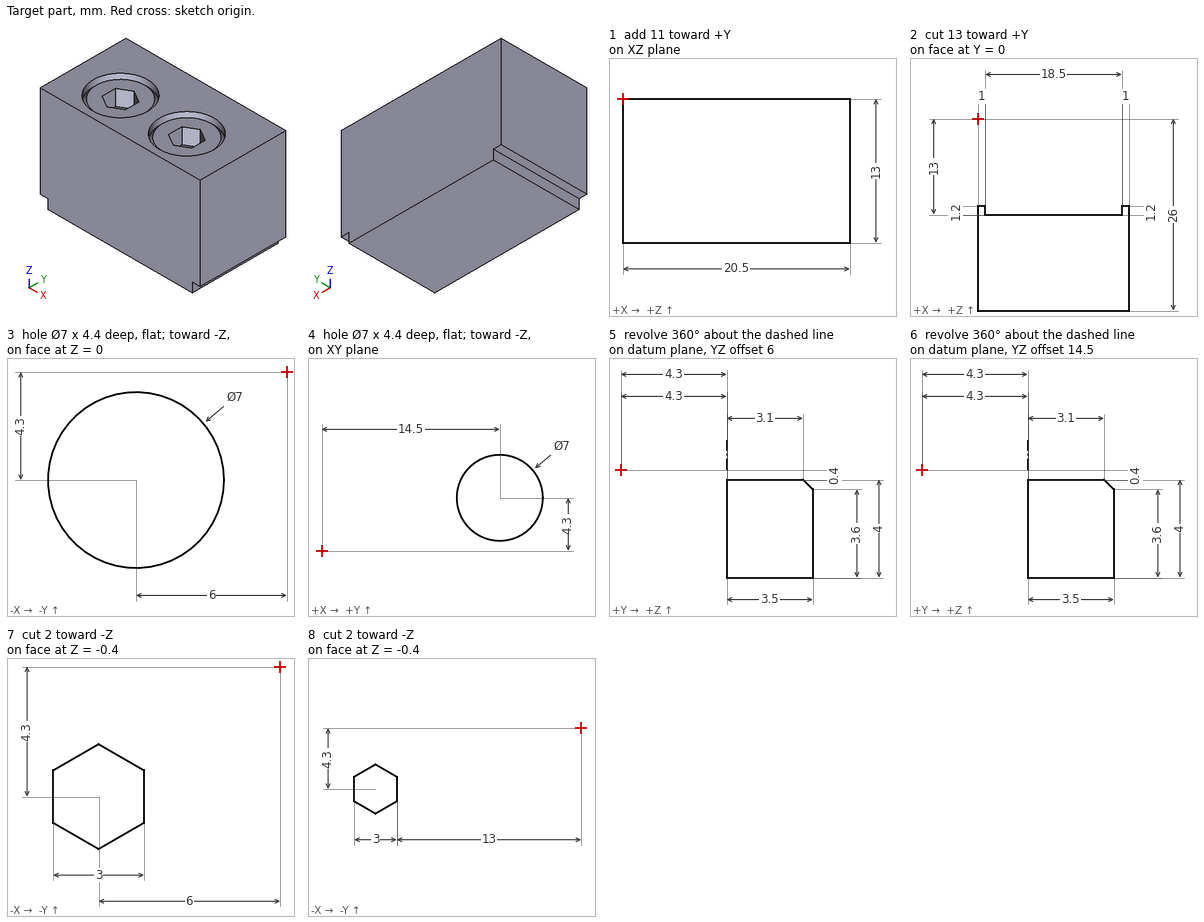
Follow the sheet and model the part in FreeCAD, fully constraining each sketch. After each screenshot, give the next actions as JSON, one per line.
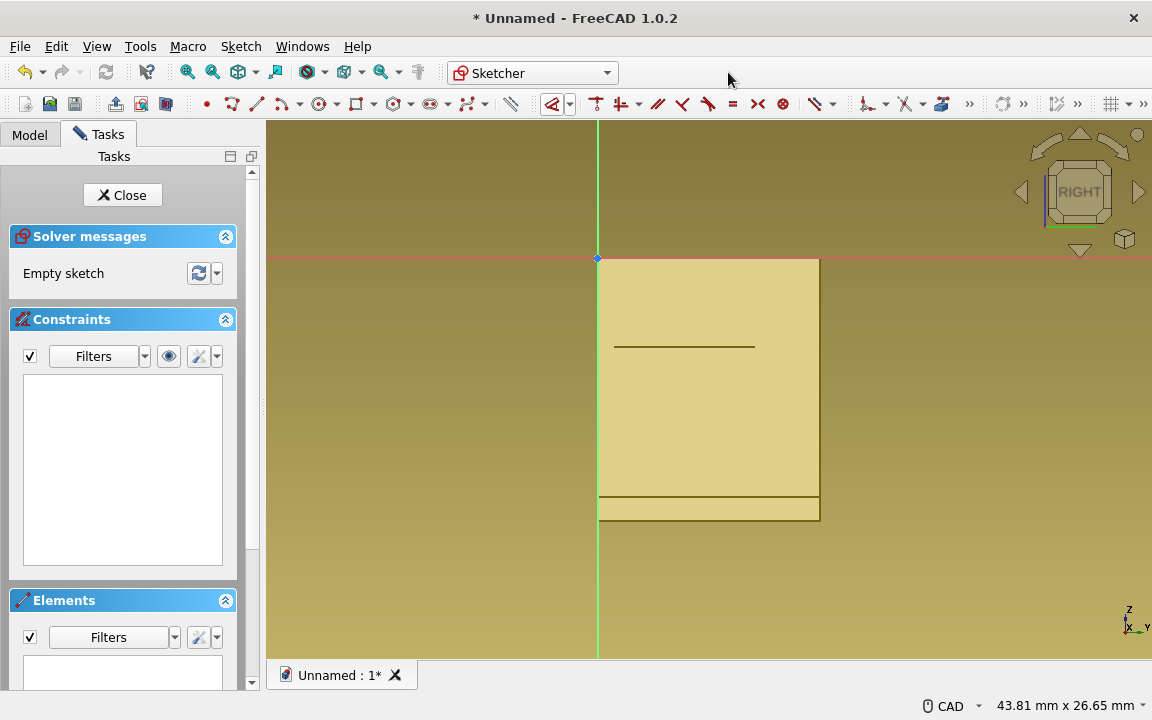
{"action": "scroll", "coordinate": [692, 248], "scroll_direction": "up", "scroll_amount": 6}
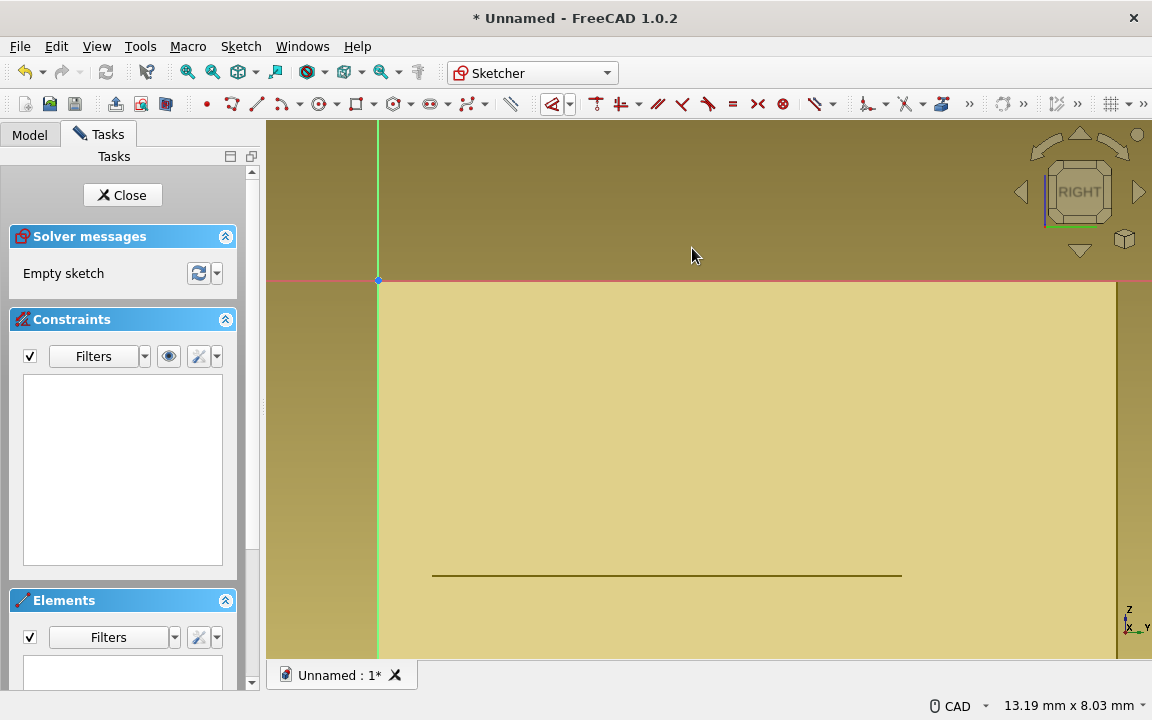
{"action": "left_click", "coordinate": [232, 104]}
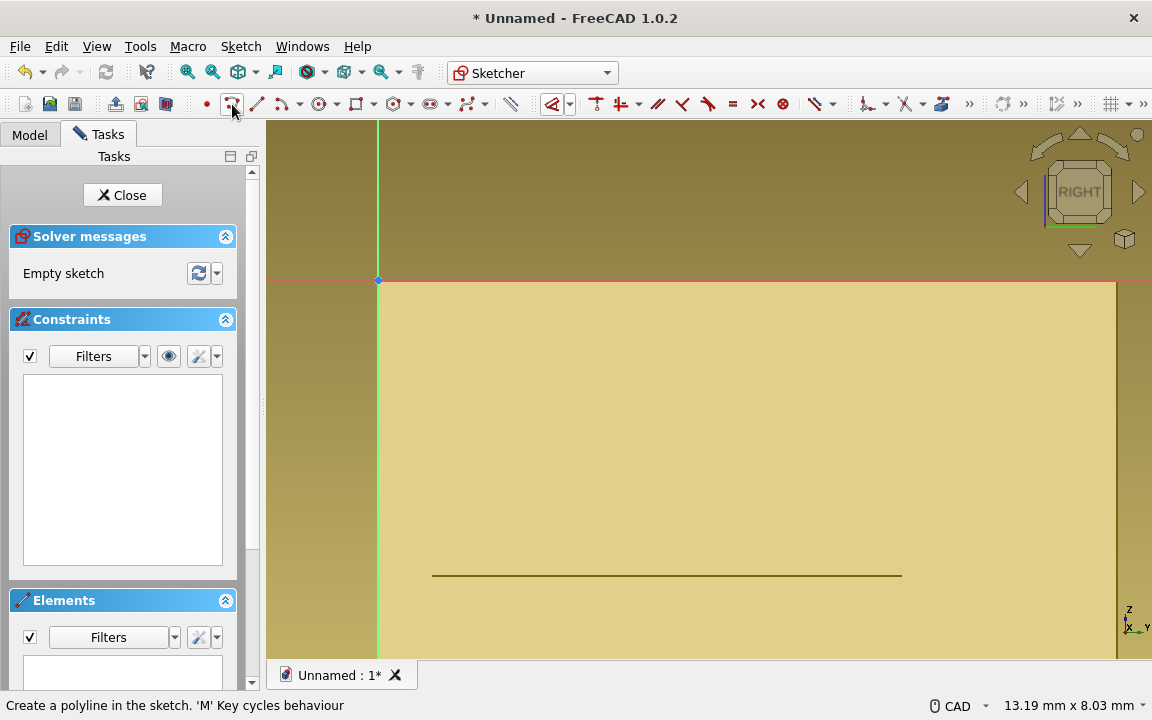
{"action": "left_click", "coordinate": [667, 308]}
{"action": "left_click", "coordinate": [667, 576]}
{"action": "left_click", "coordinate": [902, 576]}
{"action": "left_click", "coordinate": [902, 334]}
{"action": "left_click", "coordinate": [875, 308]}
{"action": "left_click", "coordinate": [667, 309]}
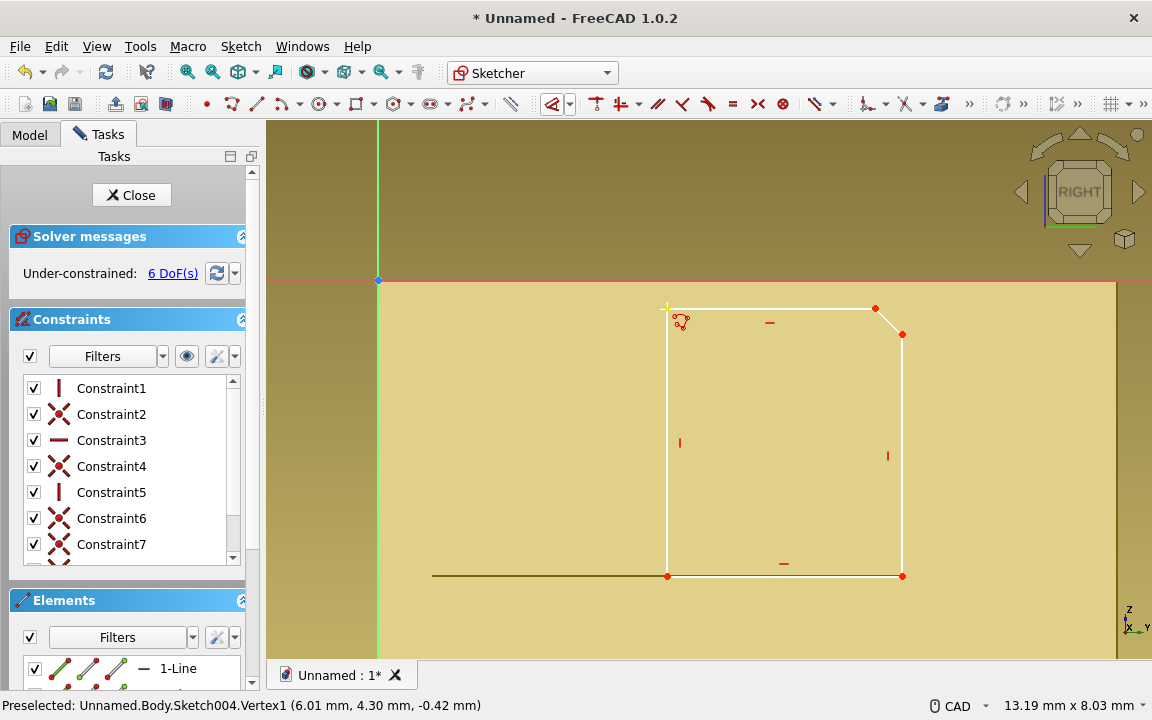
{"action": "key", "text": "g l"}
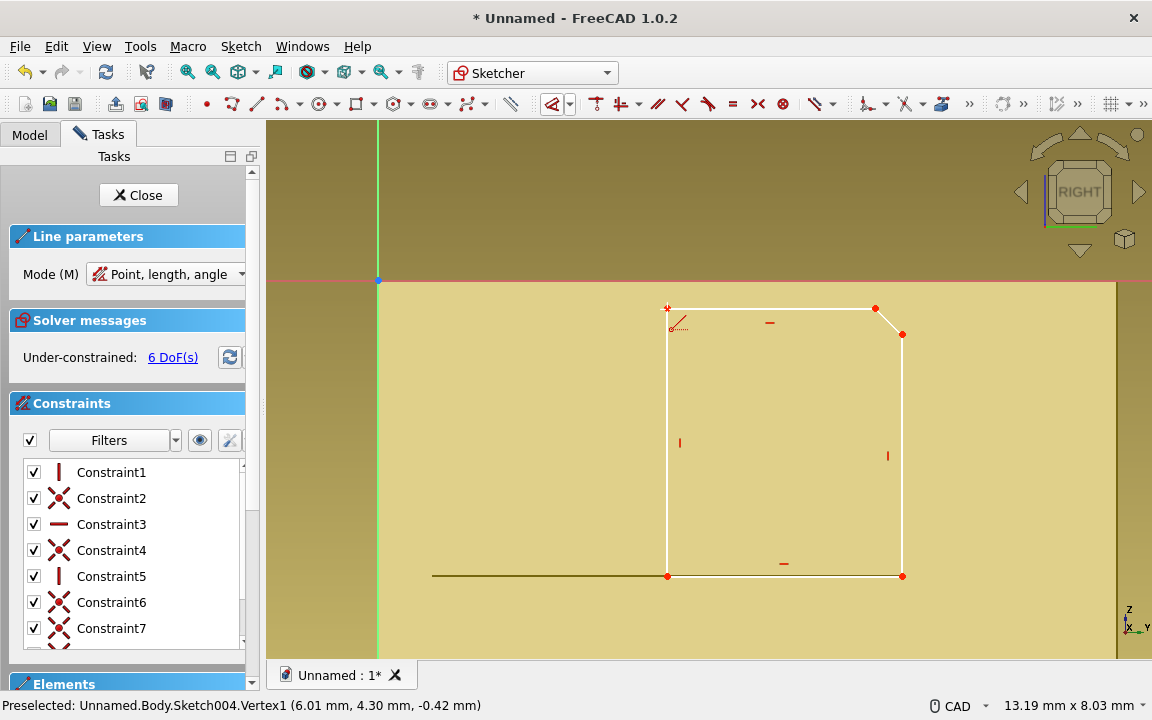
{"action": "left_click", "coordinate": [667, 281]}
{"action": "left_click", "coordinate": [667, 200]}
{"action": "key", "text": "Escape"}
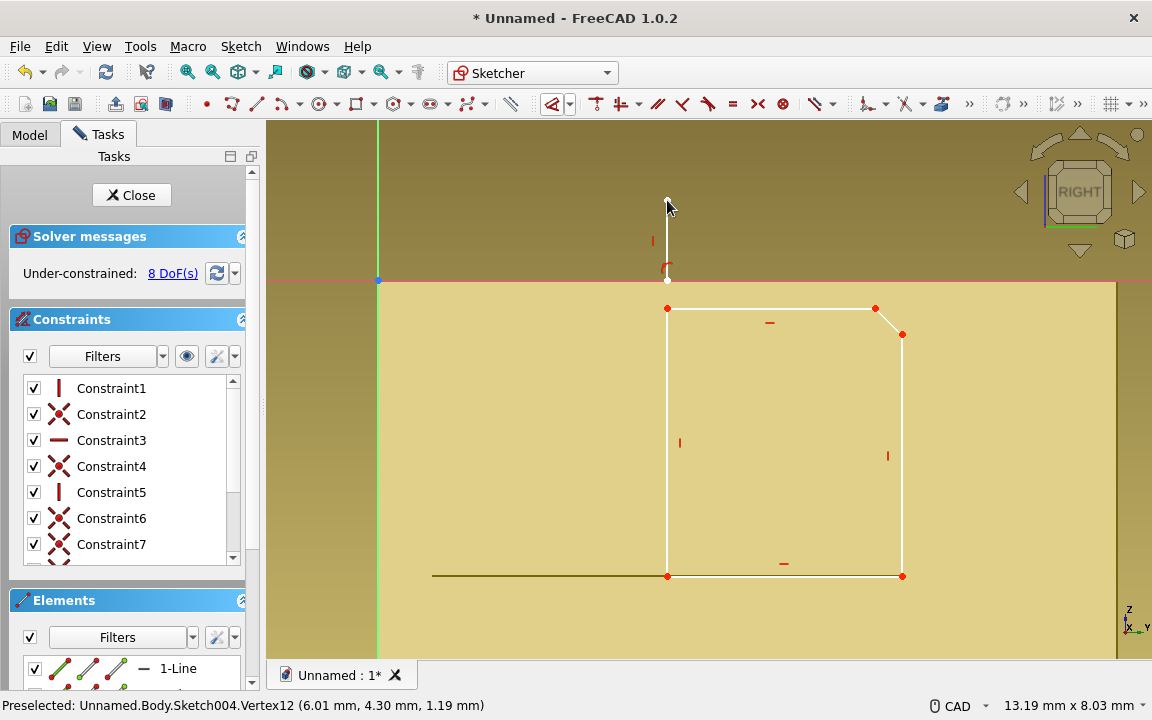
{"action": "left_click", "coordinate": [667, 257]}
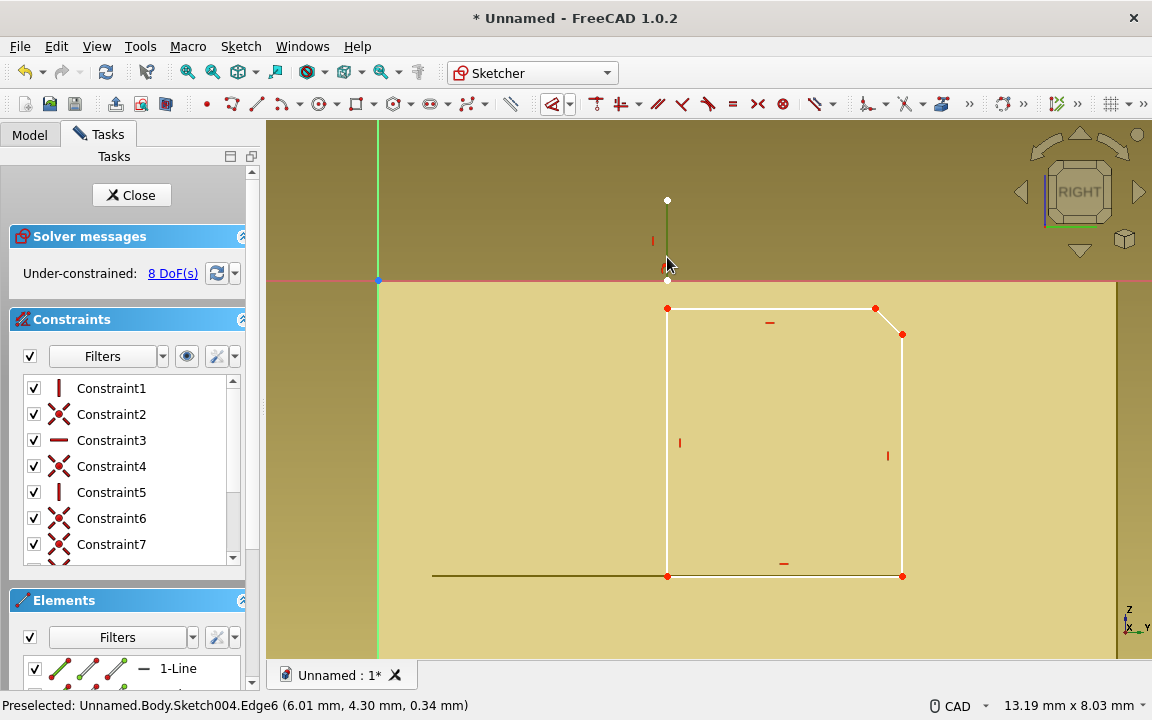
{"action": "left_click", "coordinate": [511, 104]}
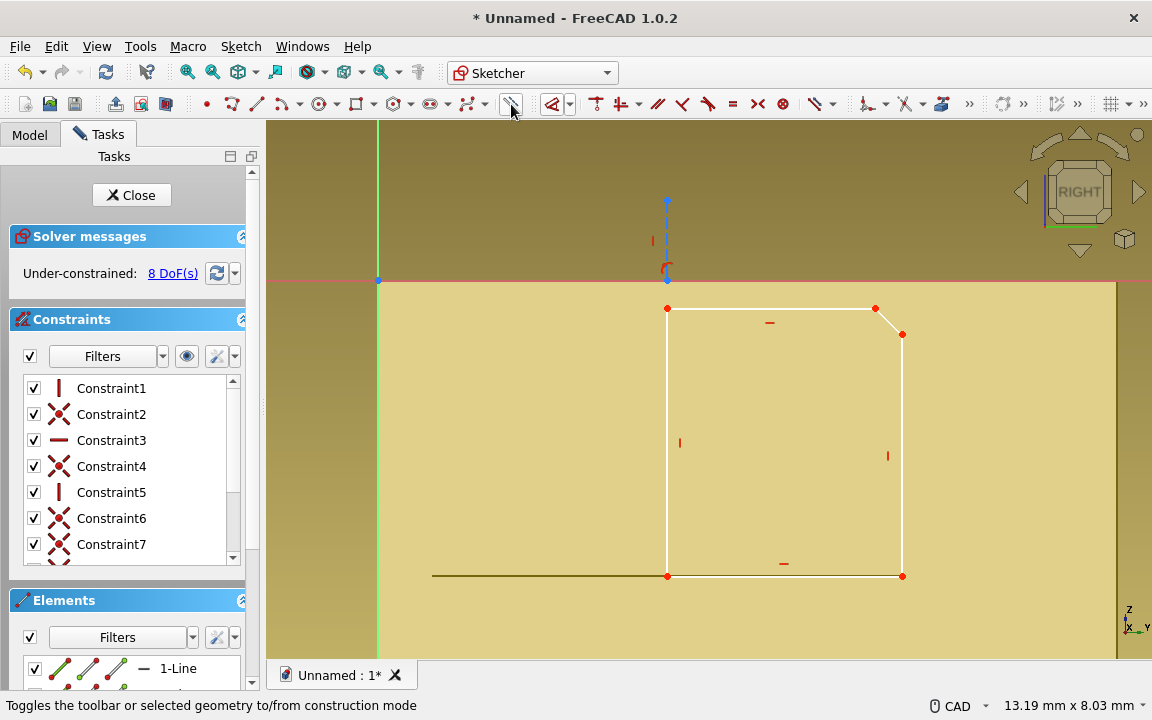
{"action": "left_click", "coordinate": [667, 389]}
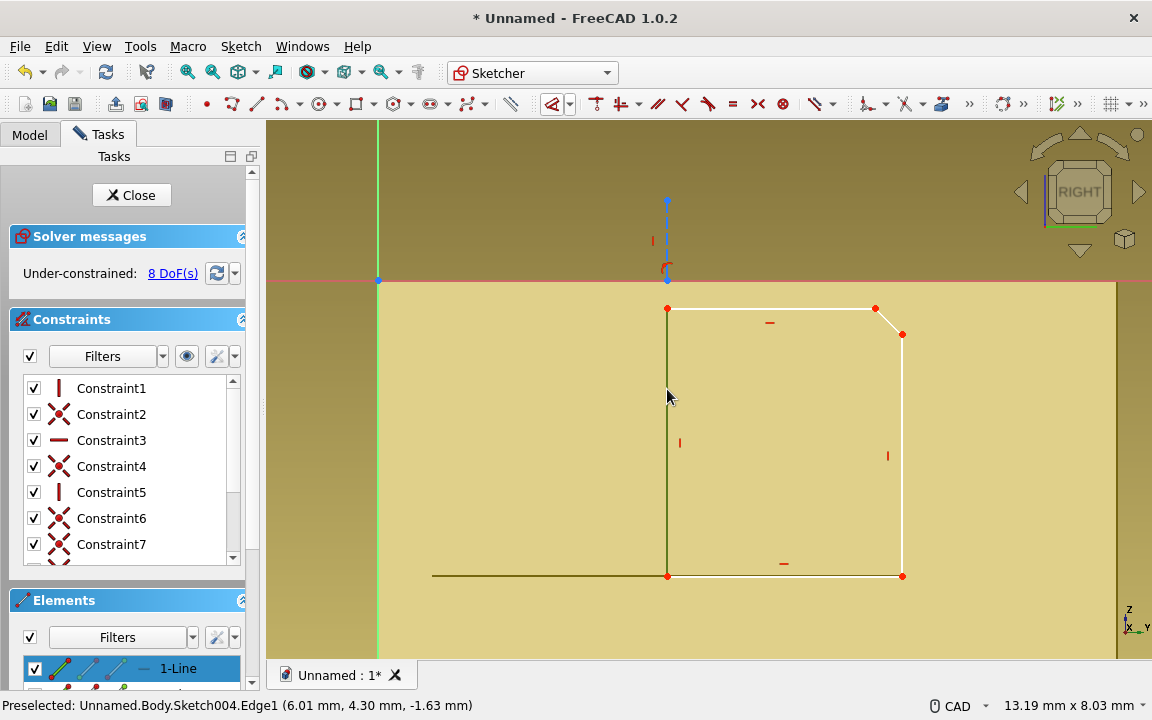
{"action": "left_click", "coordinate": [570, 104]}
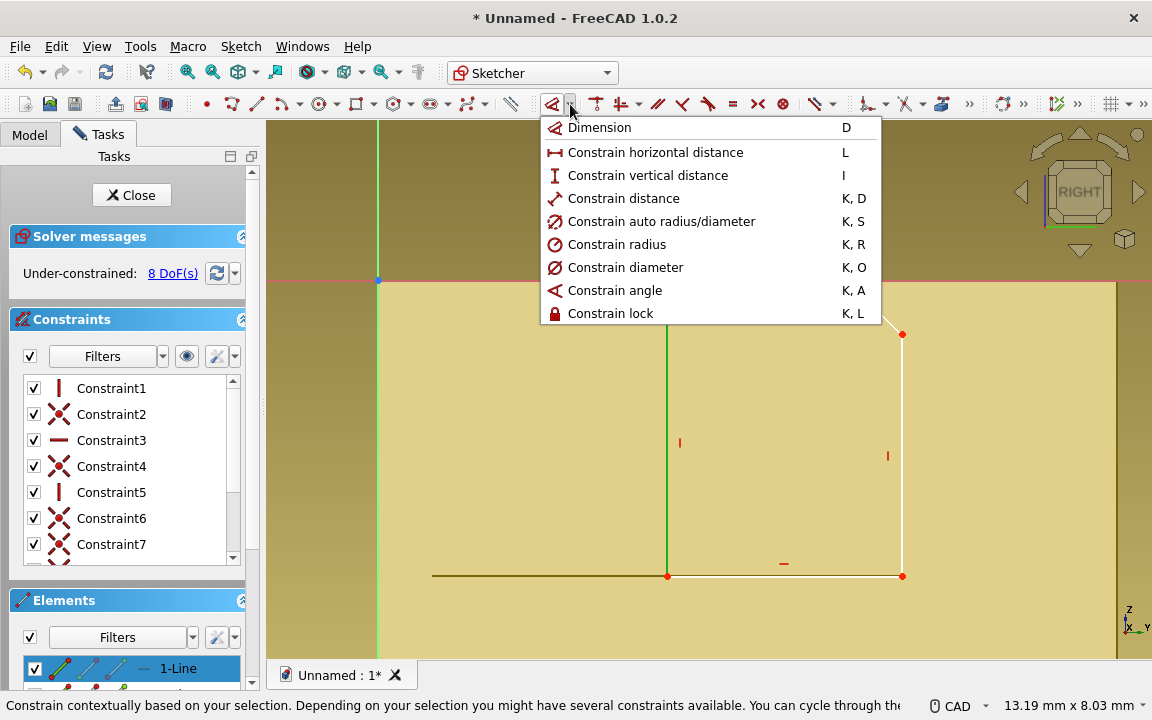
{"action": "left_click", "coordinate": [711, 176]}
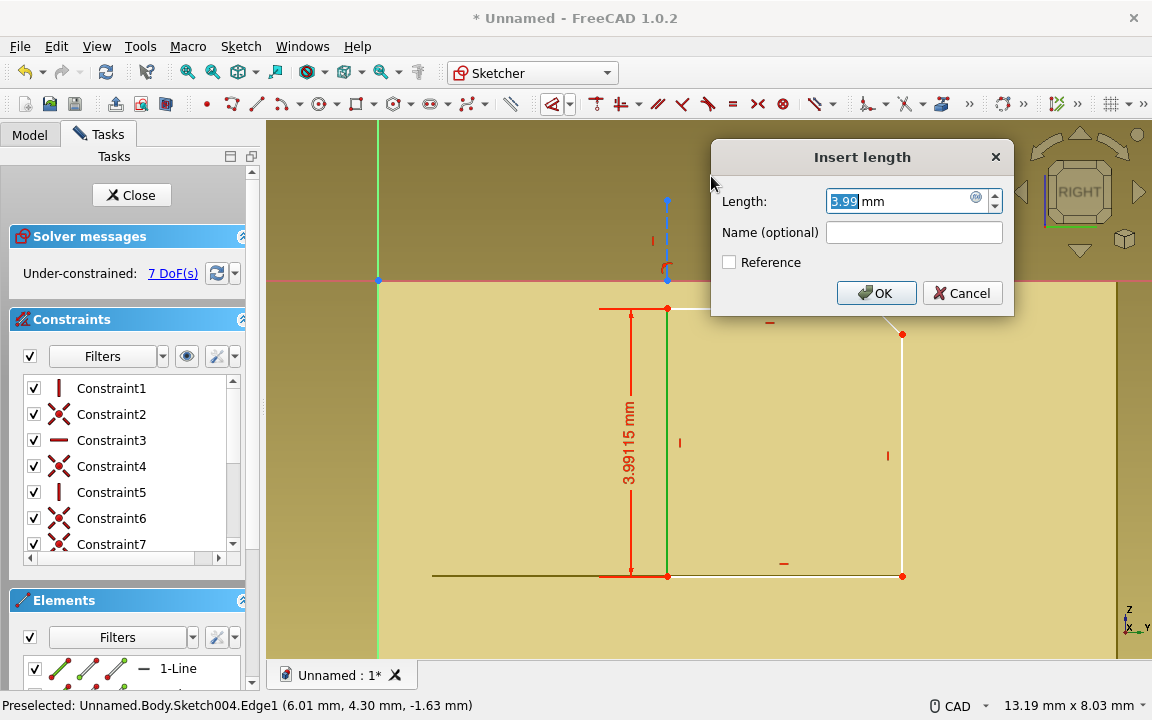
{"action": "type", "text": "4"}
{"action": "key", "text": "Return"}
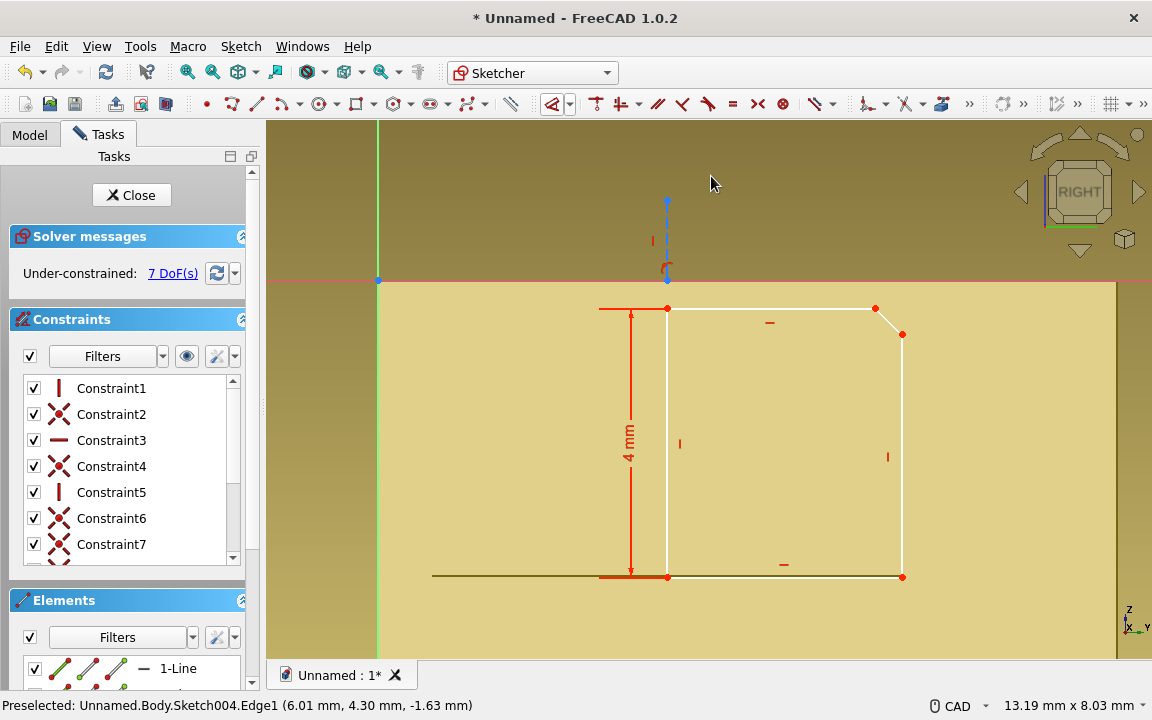
{"action": "left_click", "coordinate": [738, 578]}